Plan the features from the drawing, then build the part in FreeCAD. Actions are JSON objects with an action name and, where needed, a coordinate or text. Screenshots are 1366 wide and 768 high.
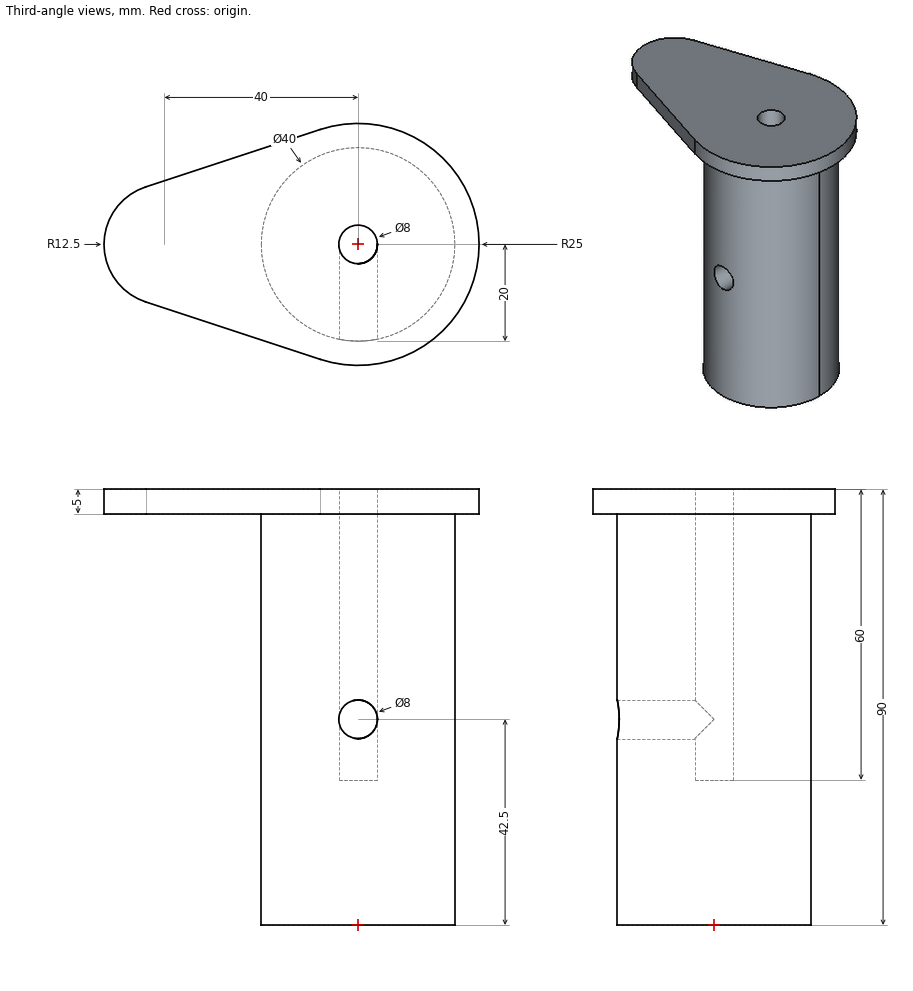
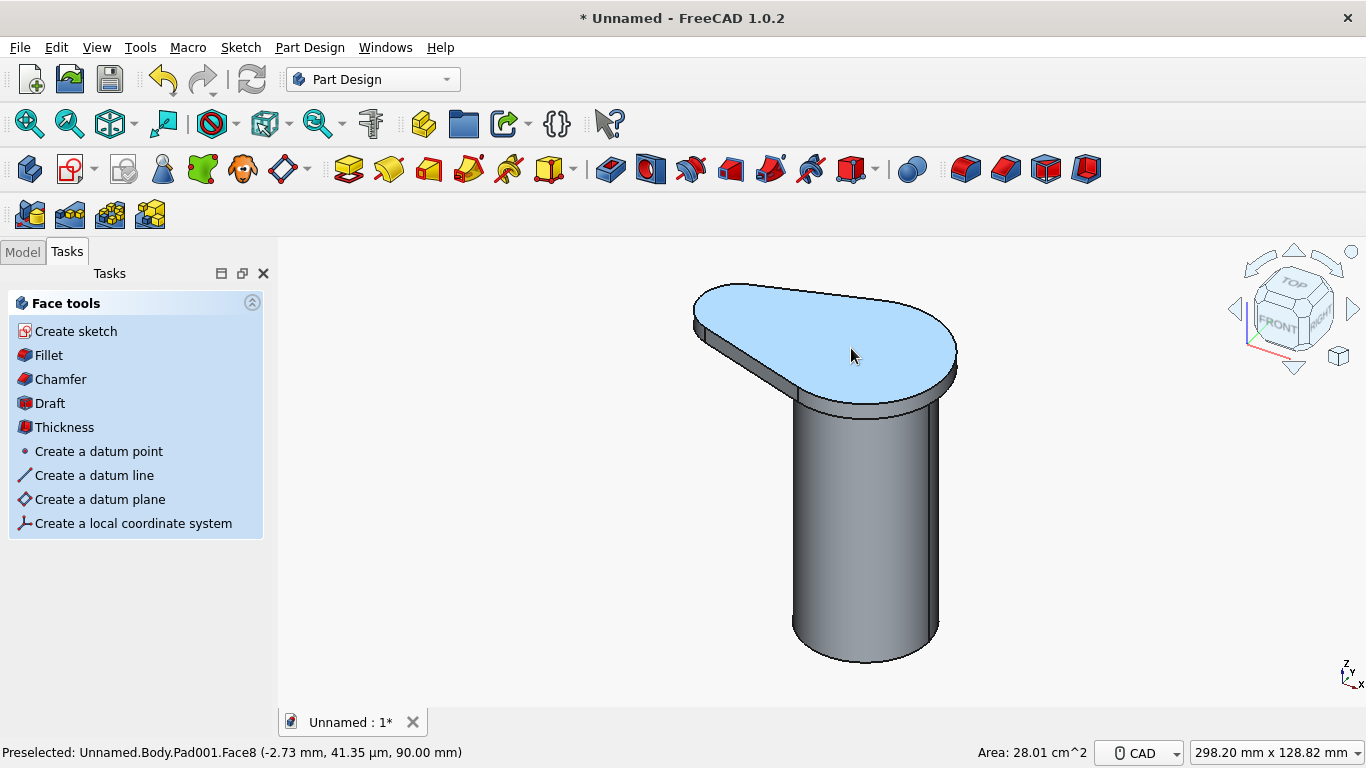
{"action": "left_click", "coordinate": [70, 170]}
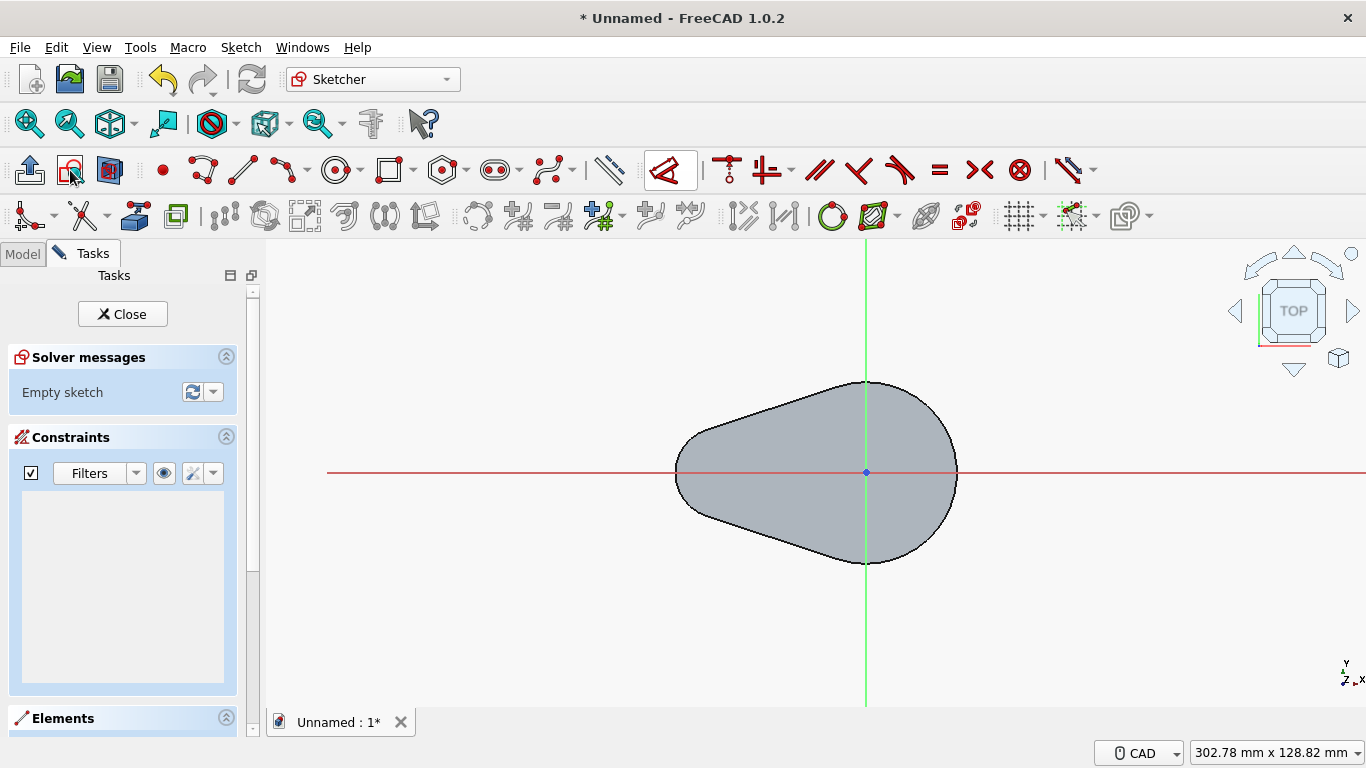
{"action": "scroll", "coordinate": [878, 473], "scroll_direction": "up", "scroll_amount": 12}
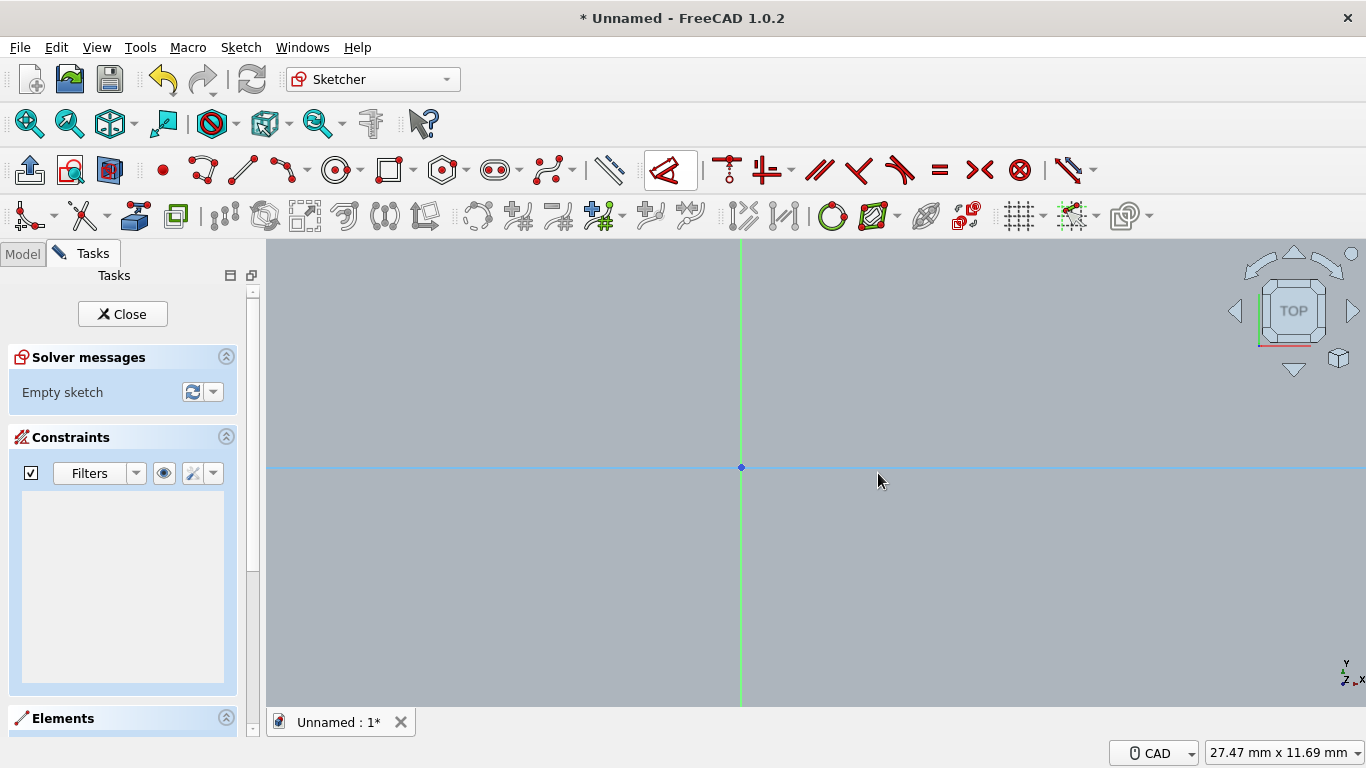
{"action": "key", "text": "g c"}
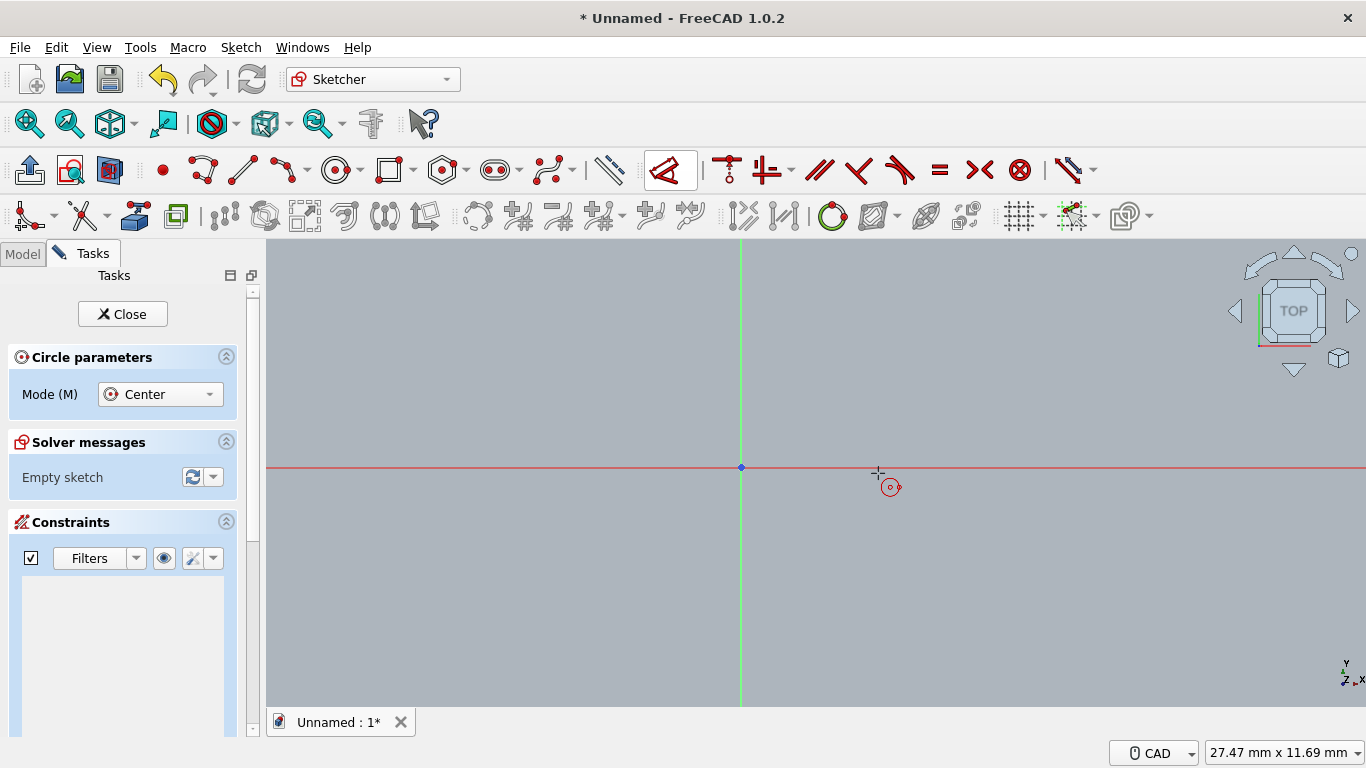
{"action": "left_click", "coordinate": [741, 468]}
{"action": "mouse_move", "coordinate": [854, 355]}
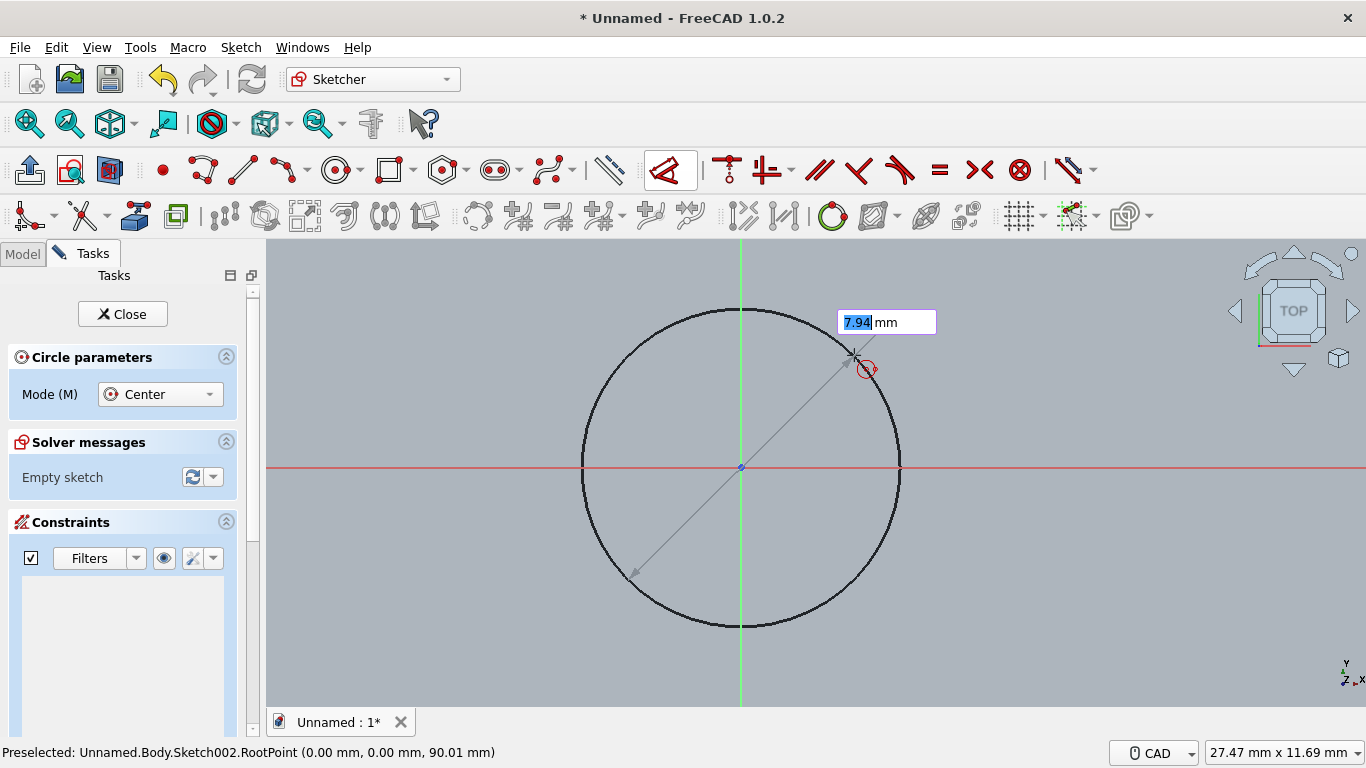
{"action": "type", "text": "8"}
{"action": "key", "text": "Return"}
{"action": "key", "text": "Escape"}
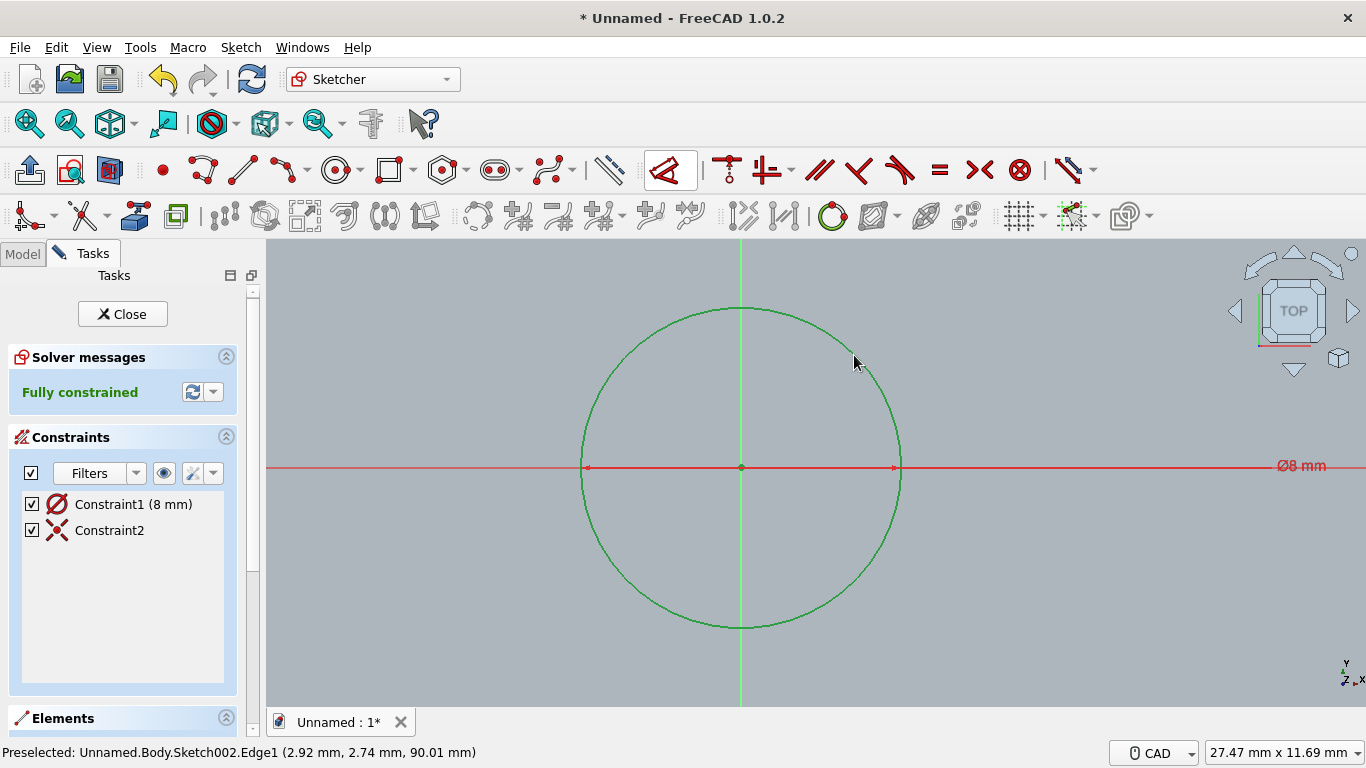
{"action": "left_click", "coordinate": [123, 314]}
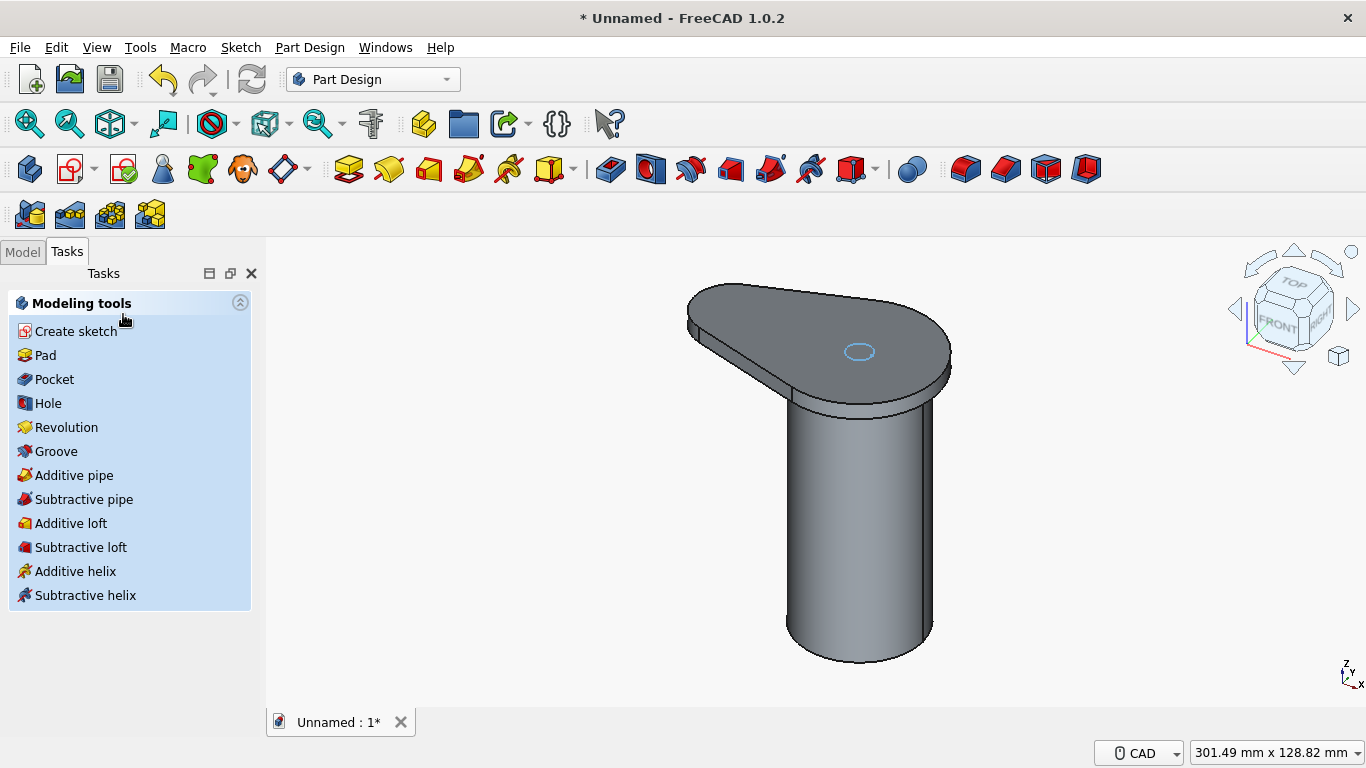
{"action": "left_click", "coordinate": [612, 170]}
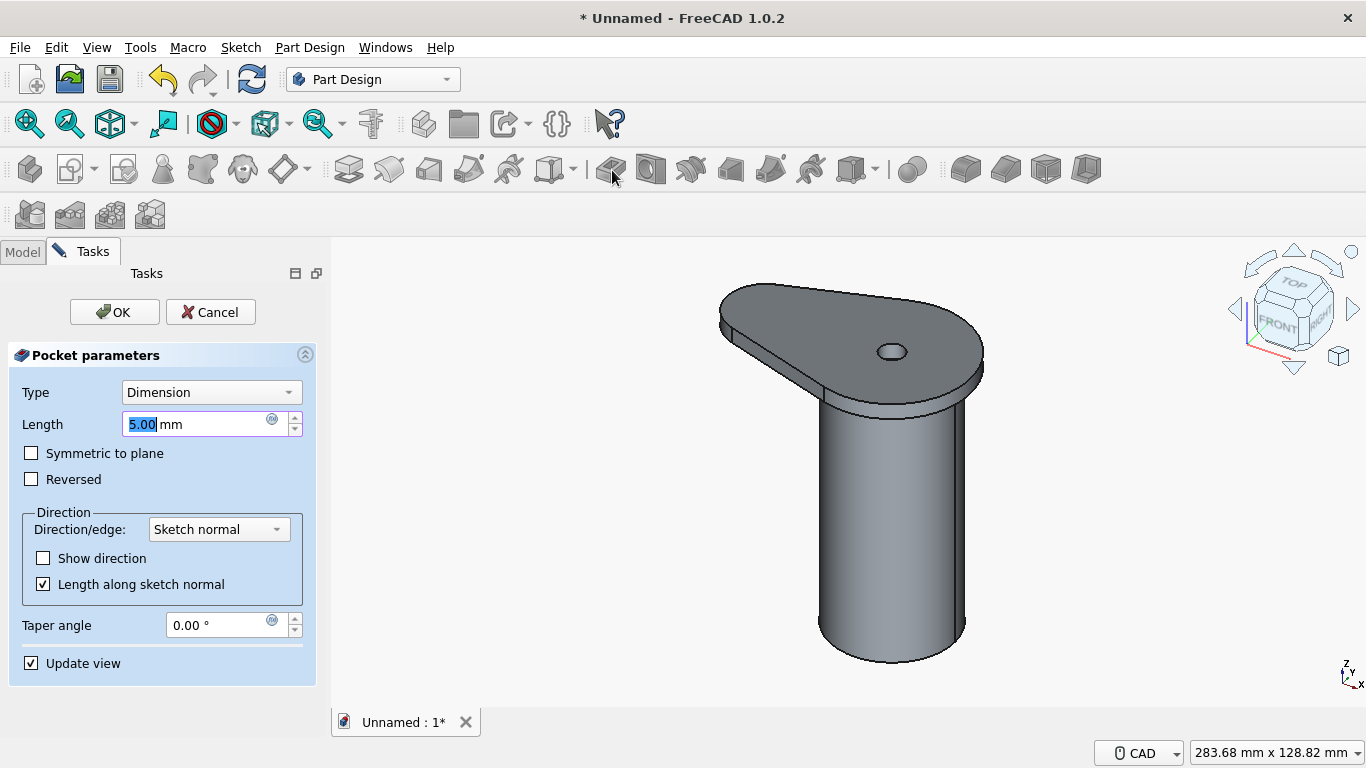
{"action": "type", "text": "60"}
{"action": "key", "text": "Tab"}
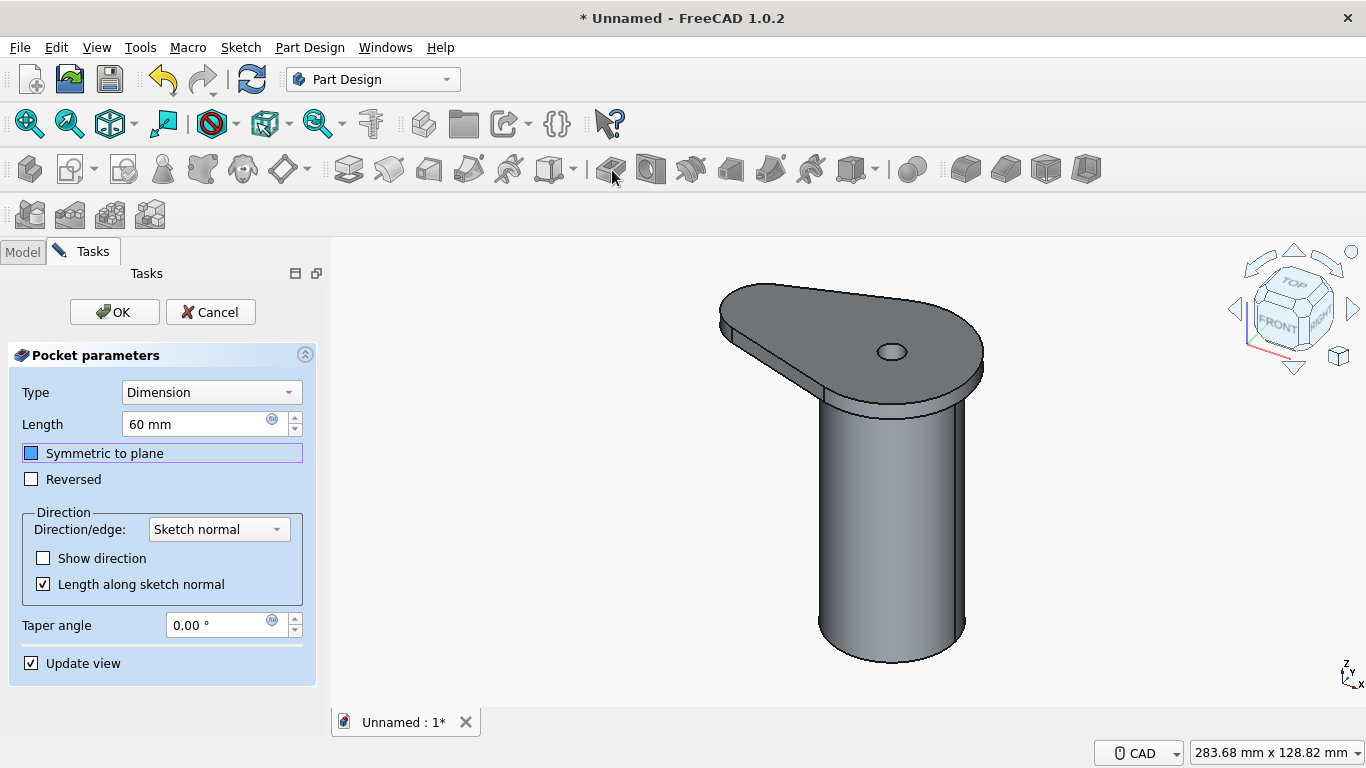
{"action": "left_click", "coordinate": [115, 312]}